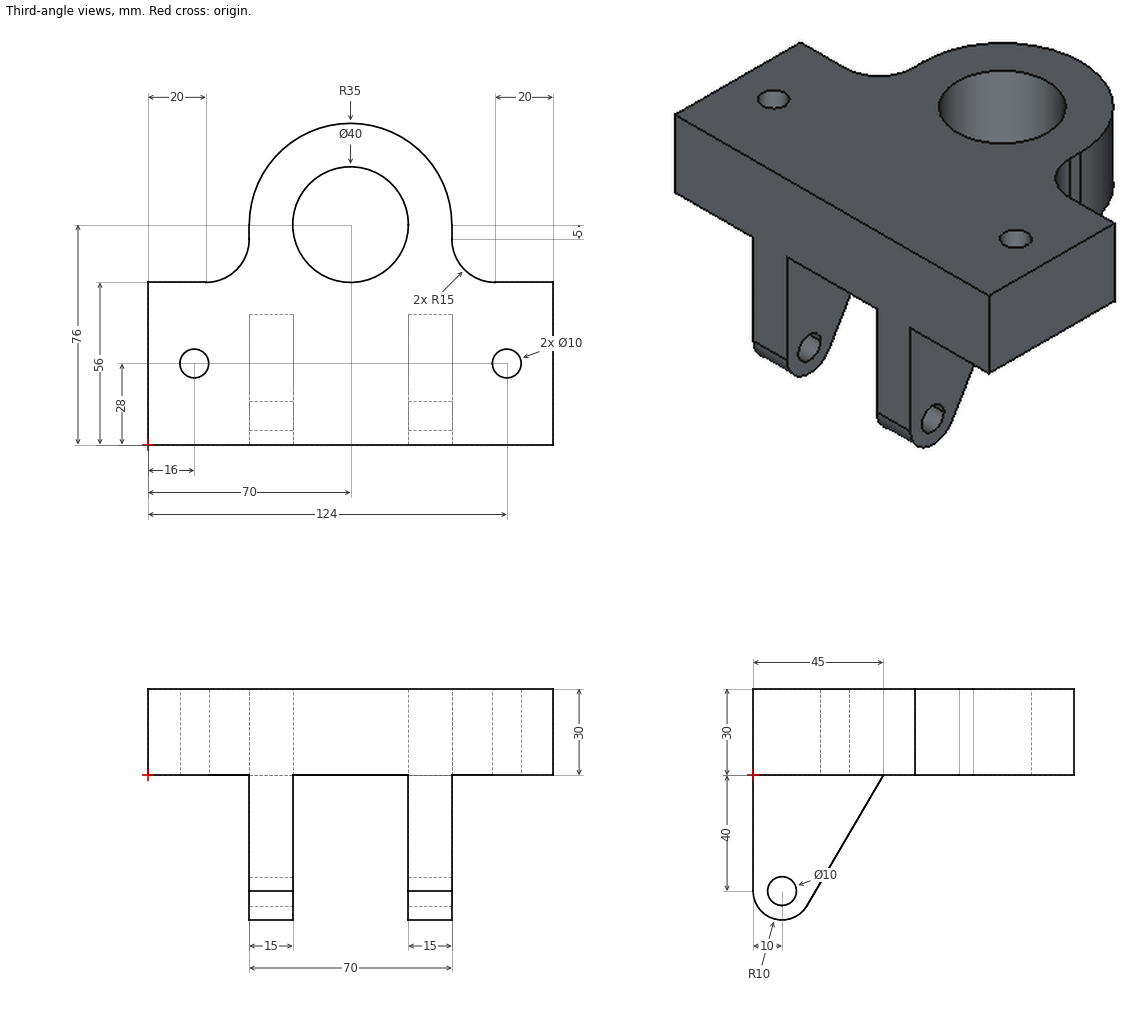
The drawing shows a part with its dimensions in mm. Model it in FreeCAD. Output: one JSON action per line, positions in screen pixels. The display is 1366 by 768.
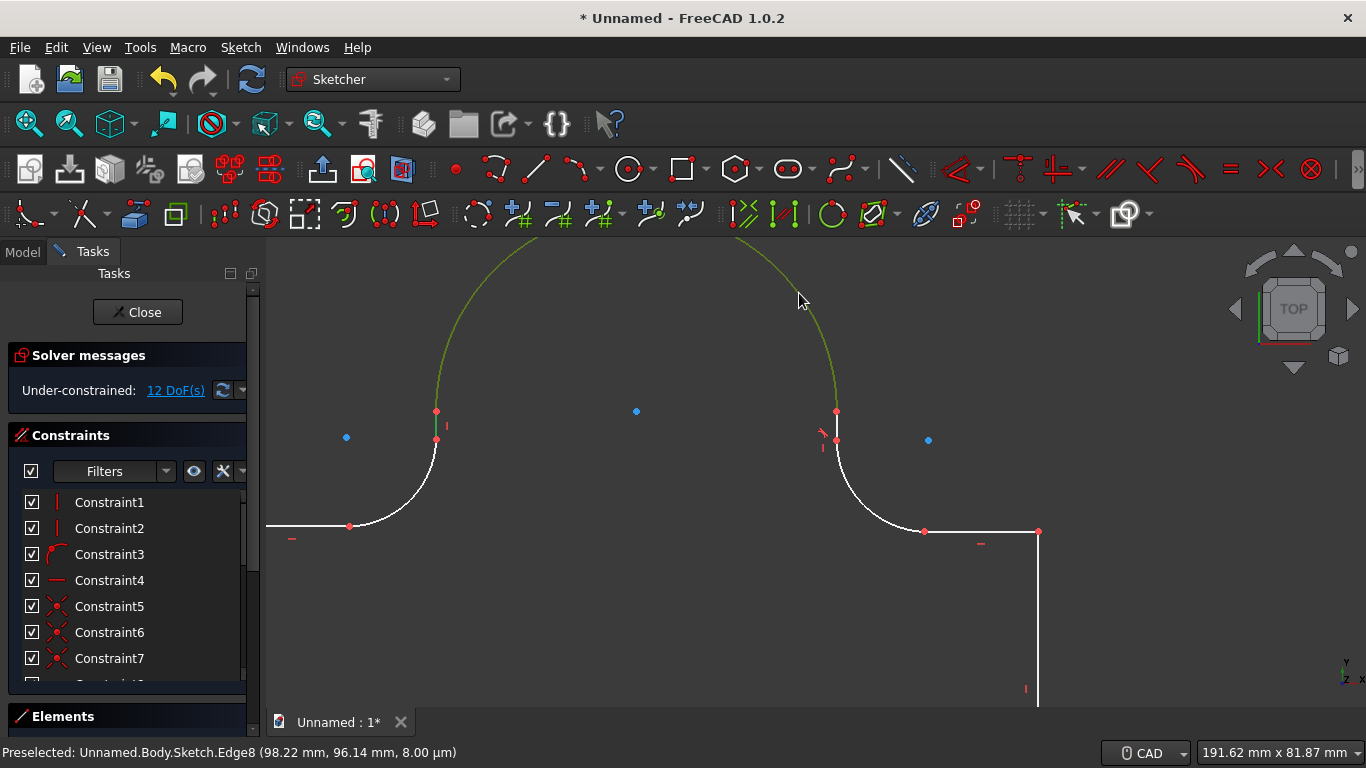
{"action": "left_click", "coordinate": [1192, 170]}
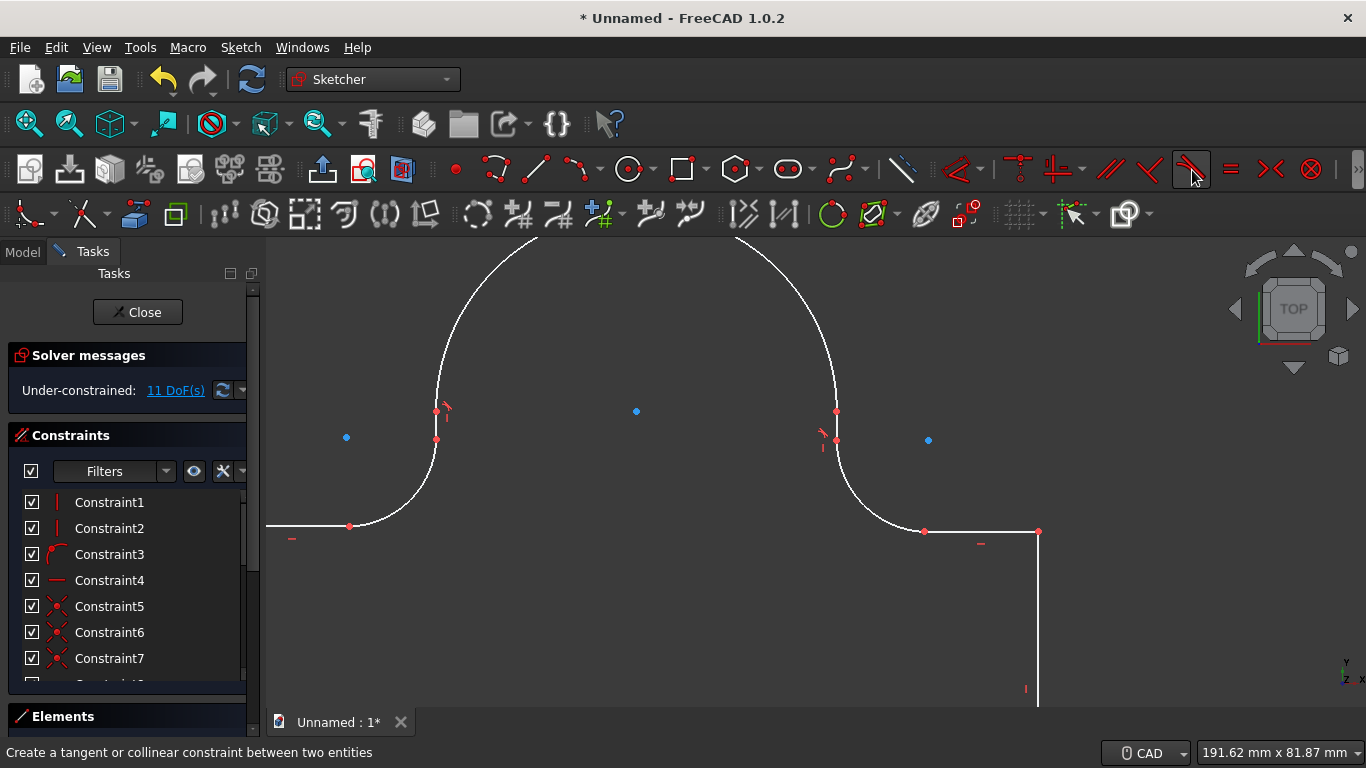
{"action": "left_click", "coordinate": [436, 423]}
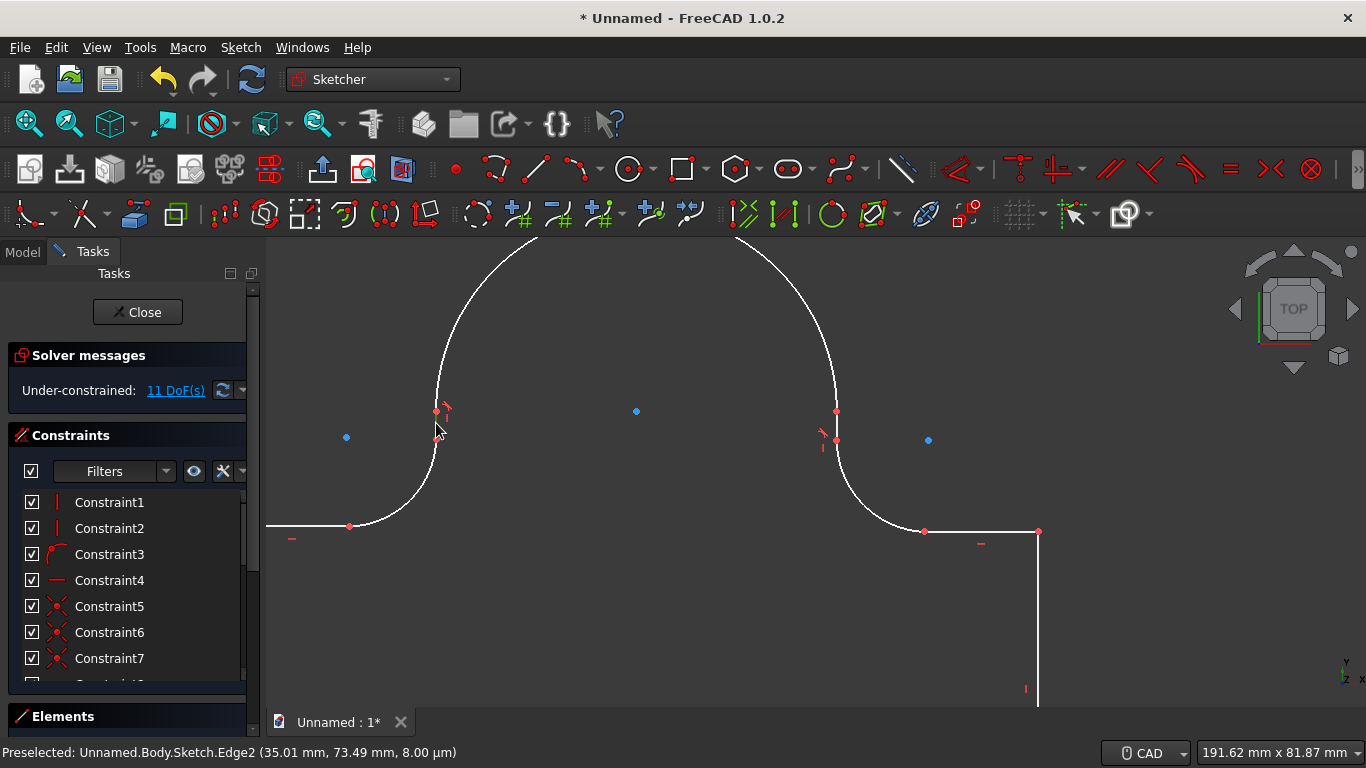
{"action": "left_click", "coordinate": [388, 516]}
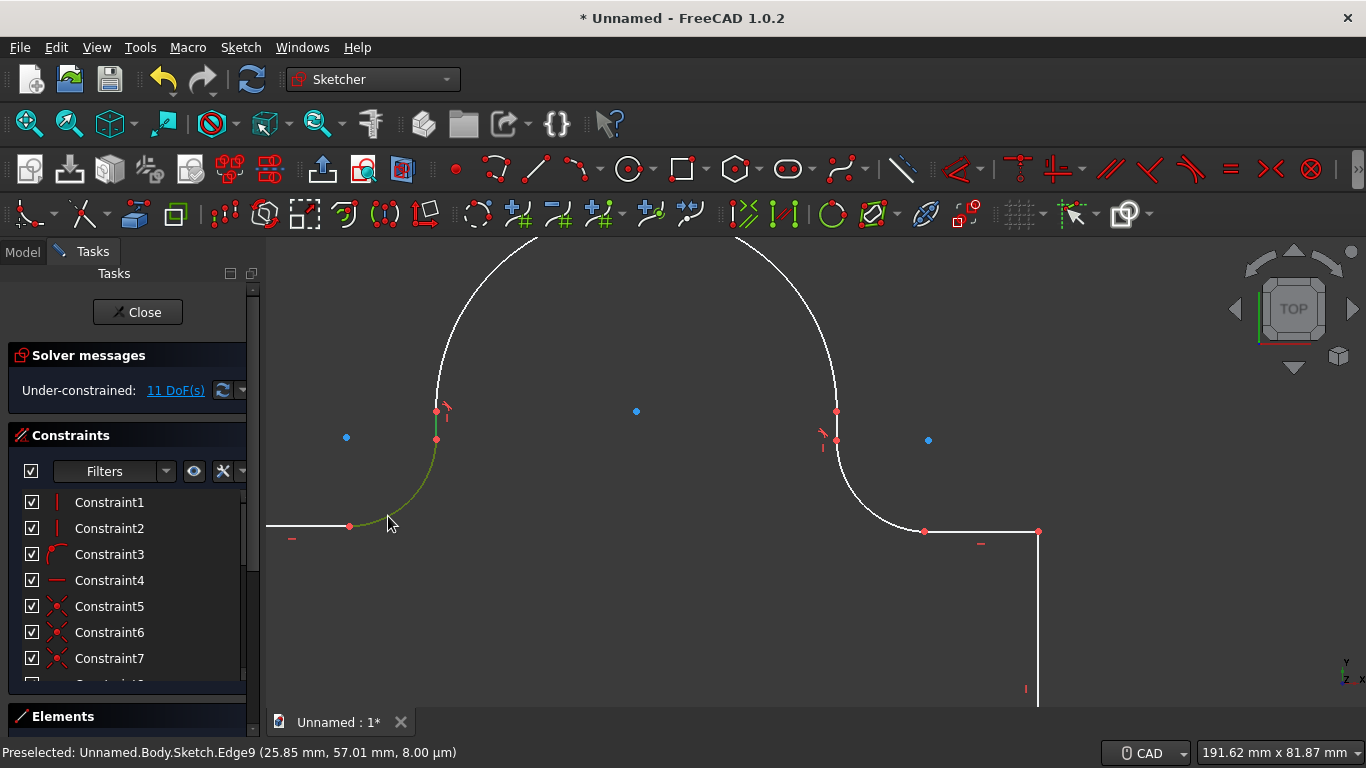
{"action": "left_click", "coordinate": [1192, 170]}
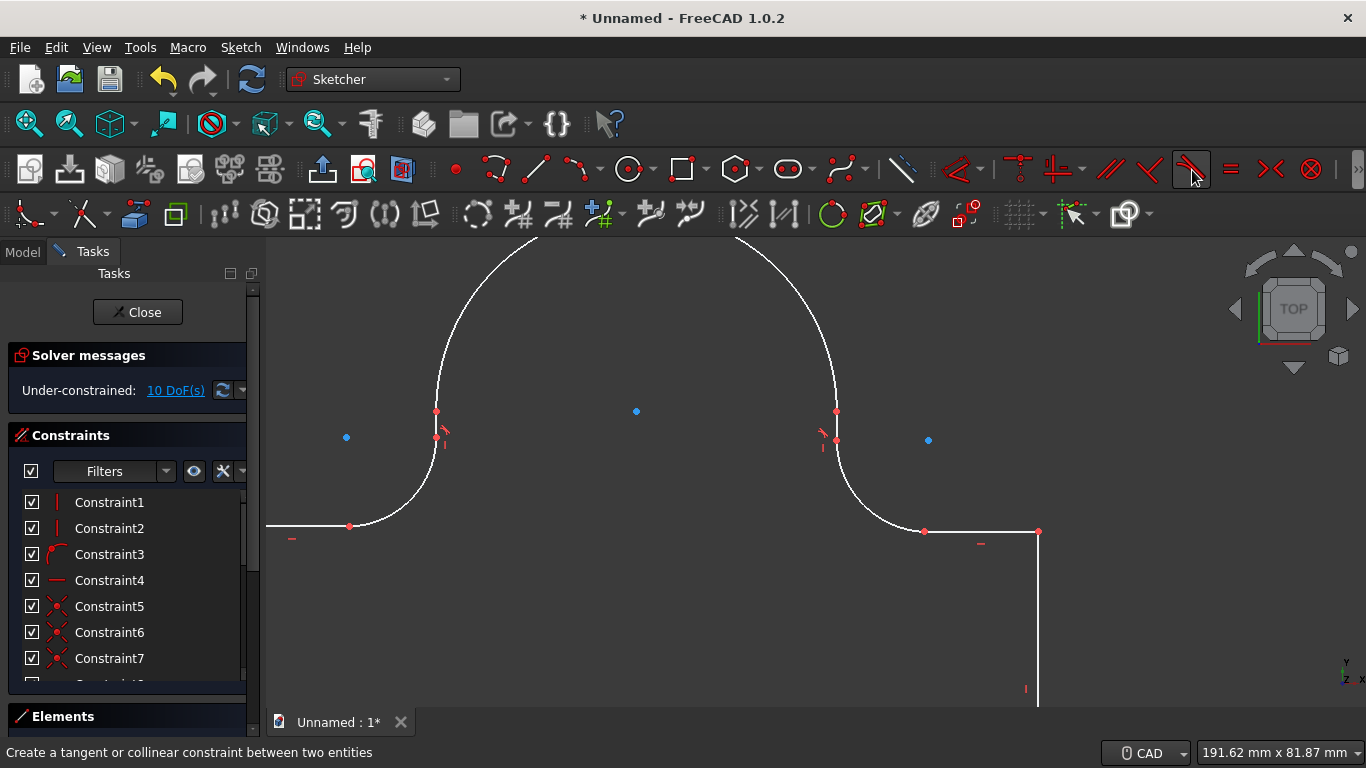
{"action": "left_click", "coordinate": [315, 526]}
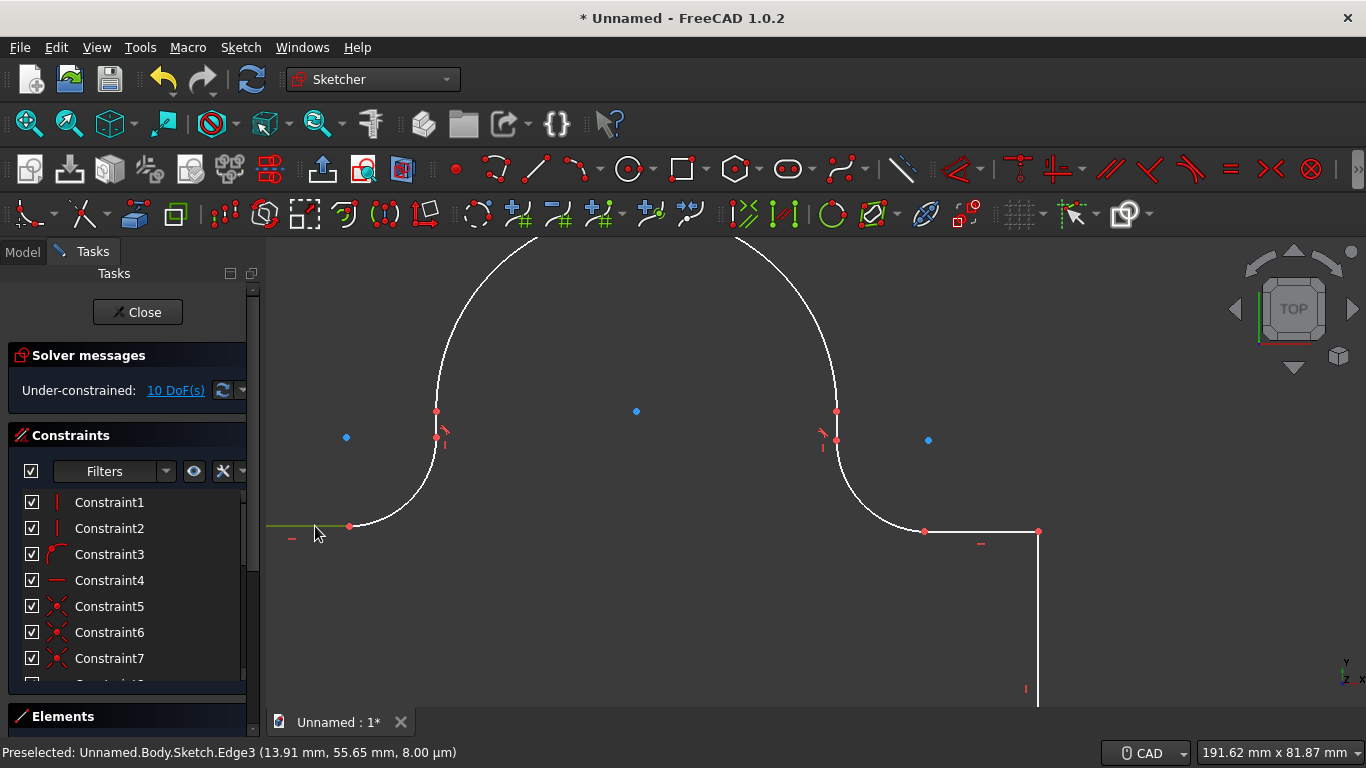
{"action": "left_click", "coordinate": [389, 516]}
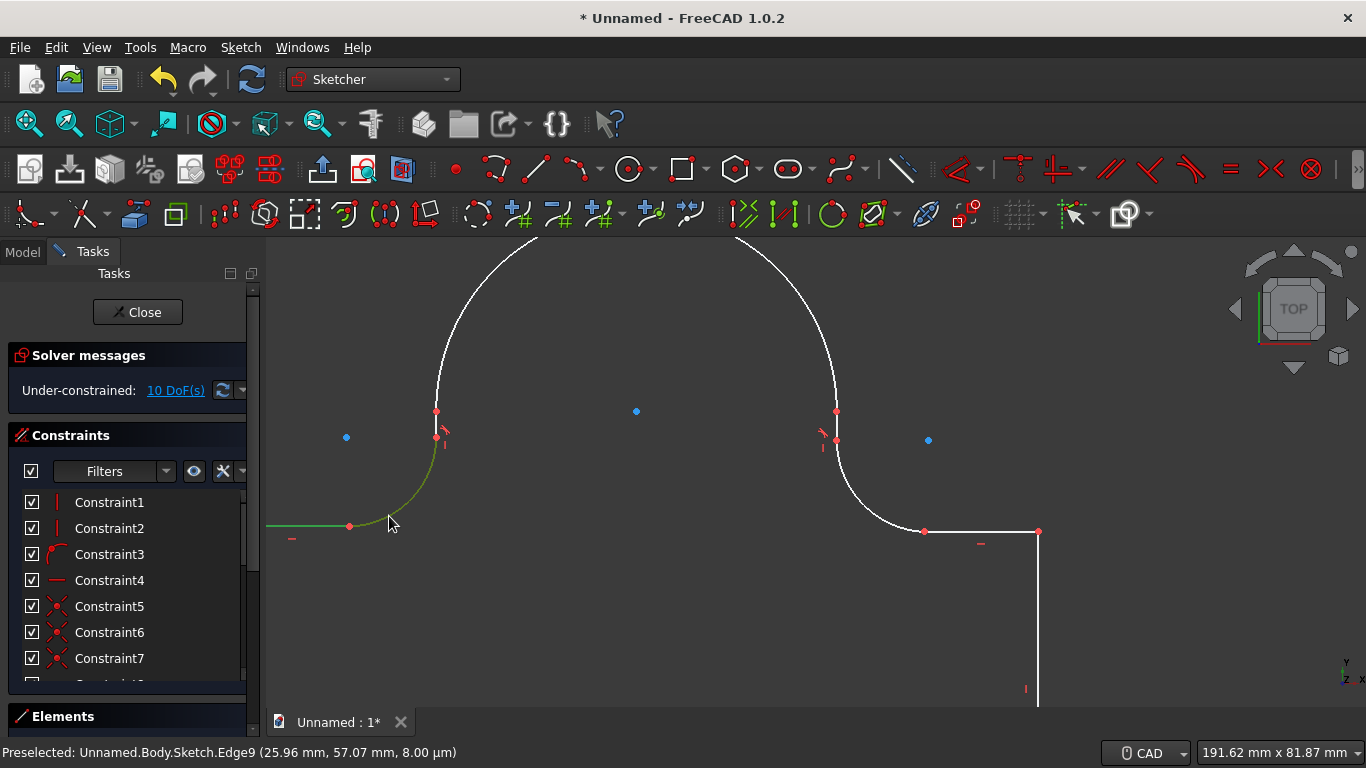
{"action": "left_click", "coordinate": [1192, 170]}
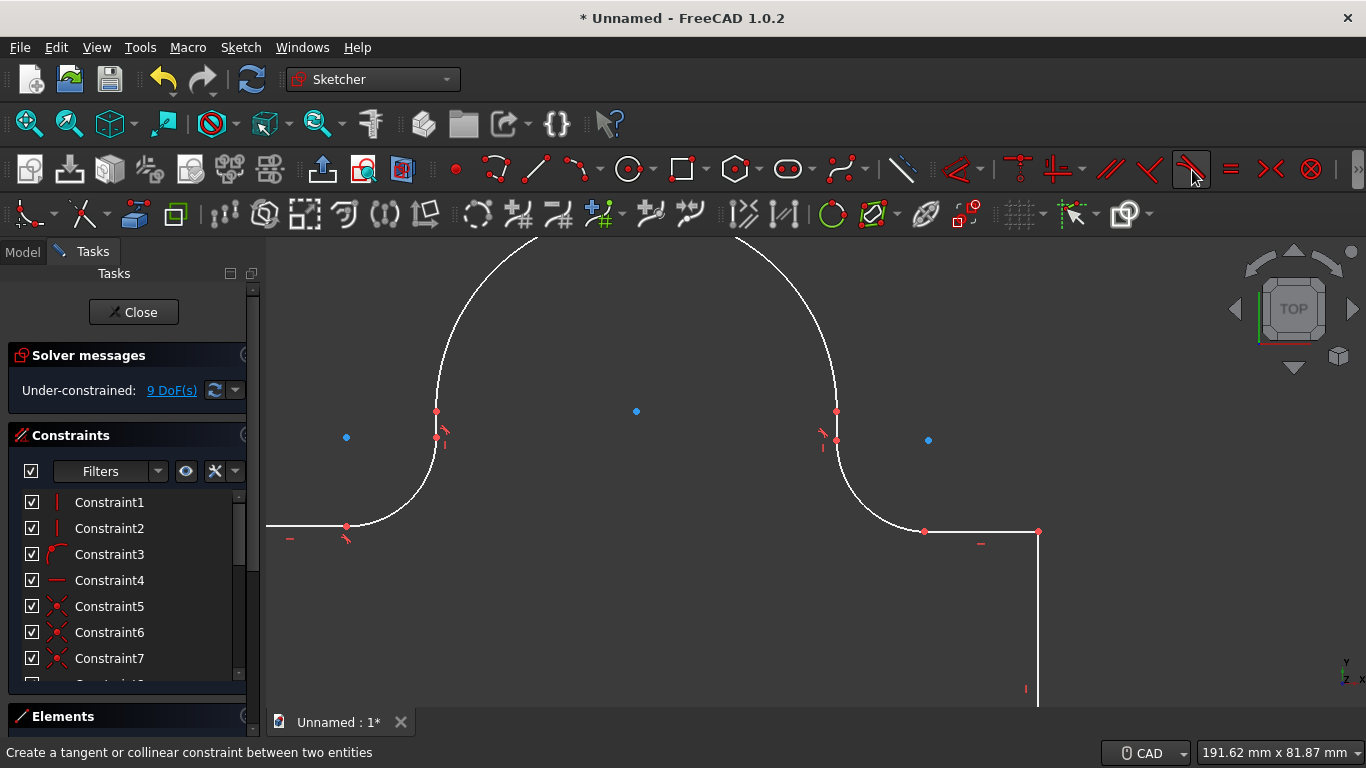
{"action": "left_click", "coordinate": [1004, 532]}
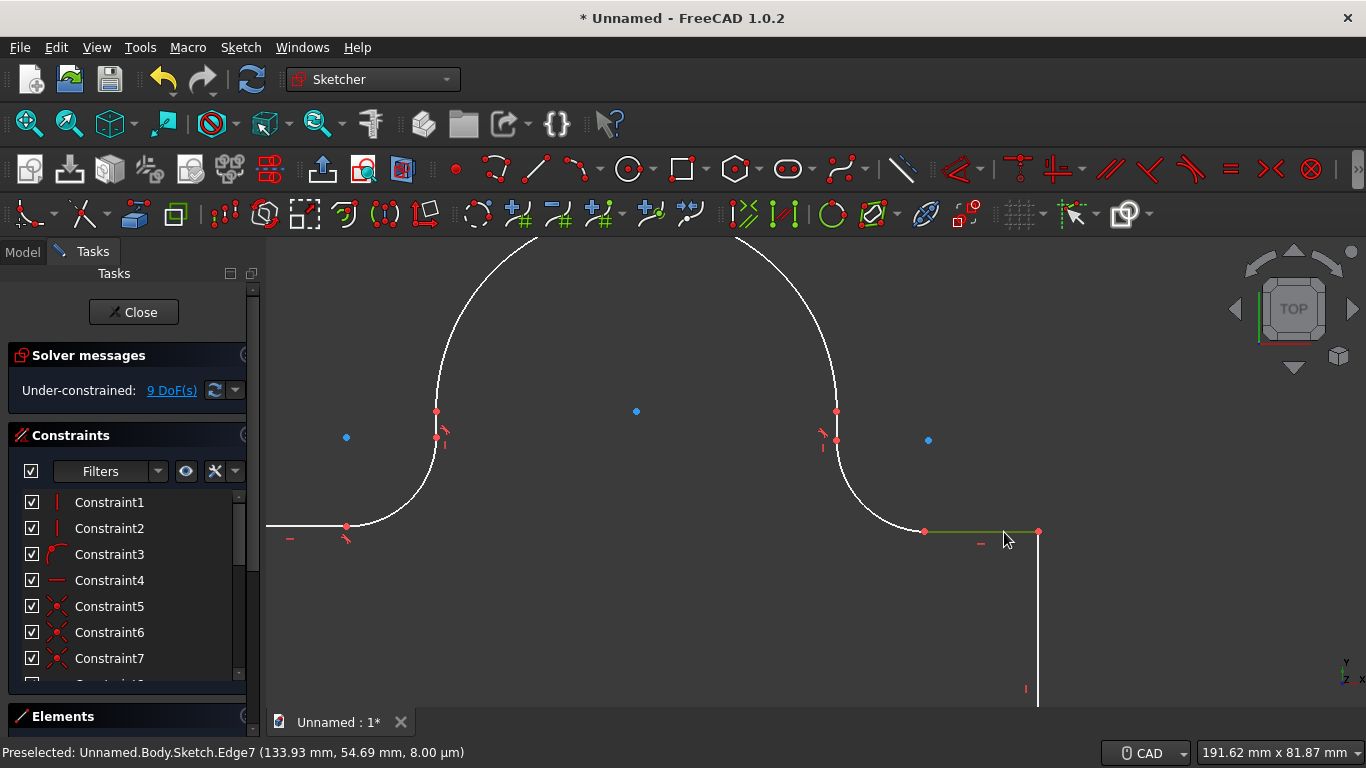
{"action": "left_click", "coordinate": [846, 481]}